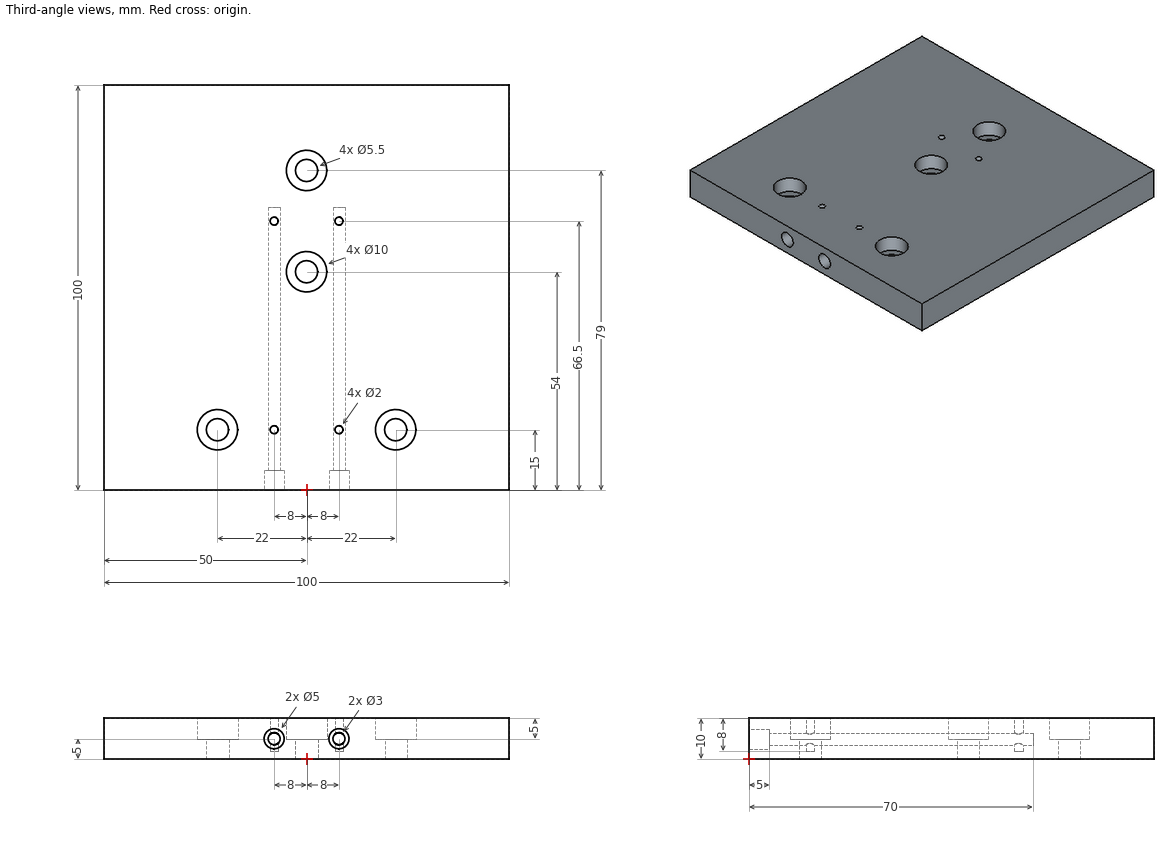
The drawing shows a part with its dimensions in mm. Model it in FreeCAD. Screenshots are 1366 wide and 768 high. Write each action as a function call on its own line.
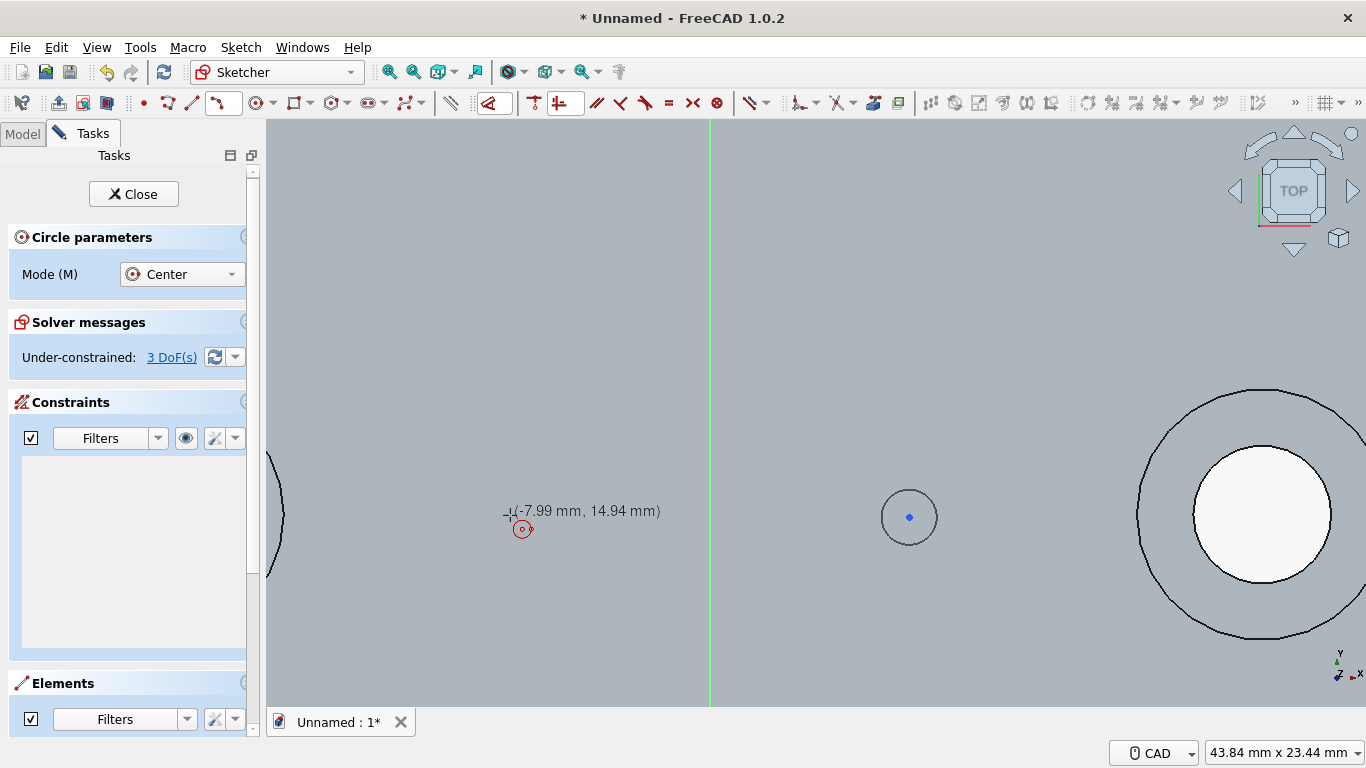
scroll(757, 506, down, 8)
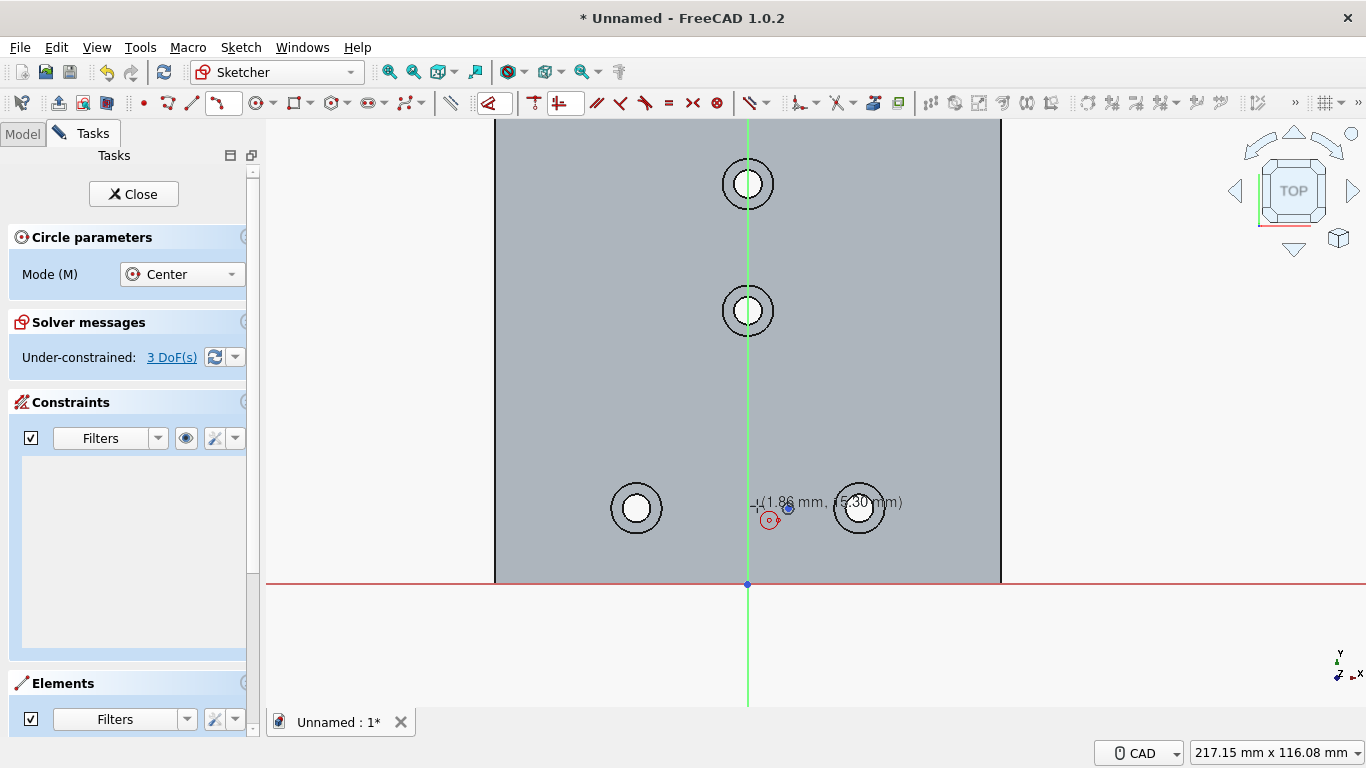
click(707, 508)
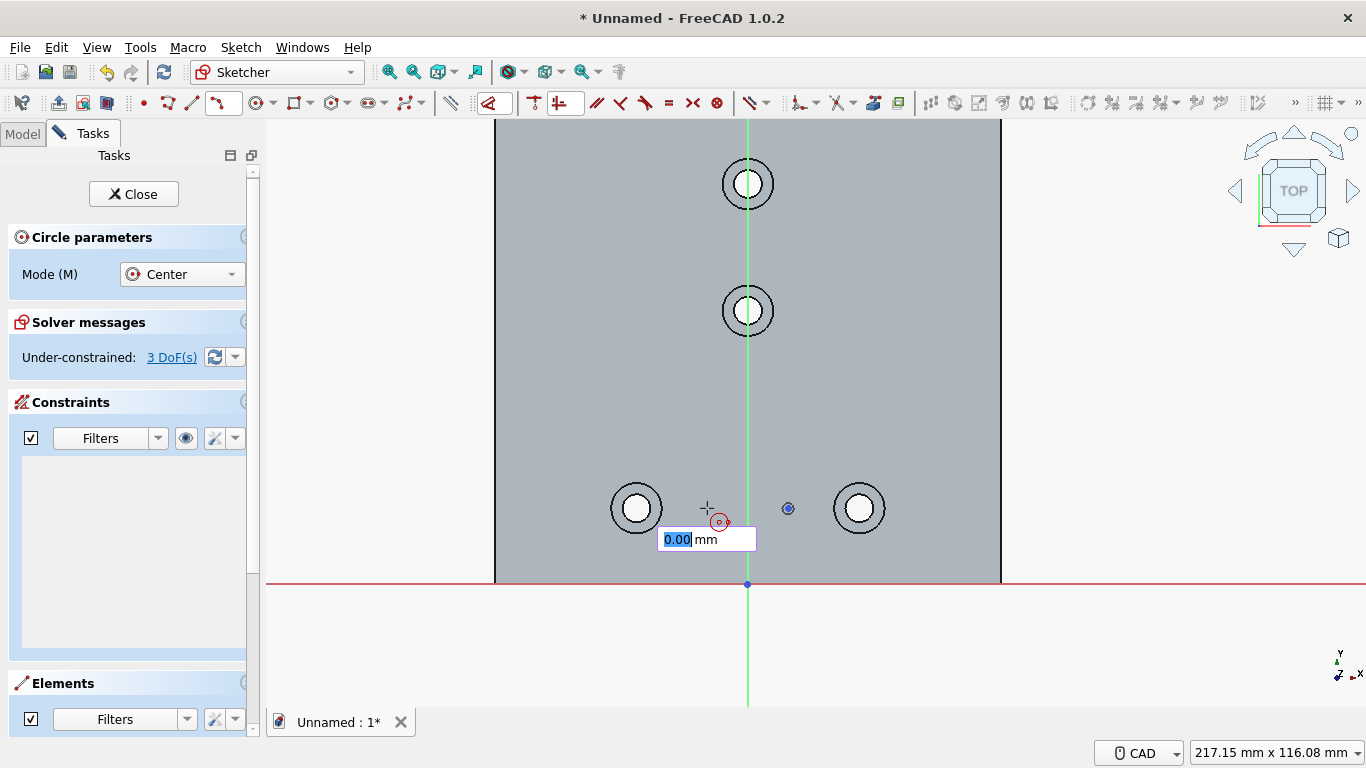
scroll(711, 505, up, 6)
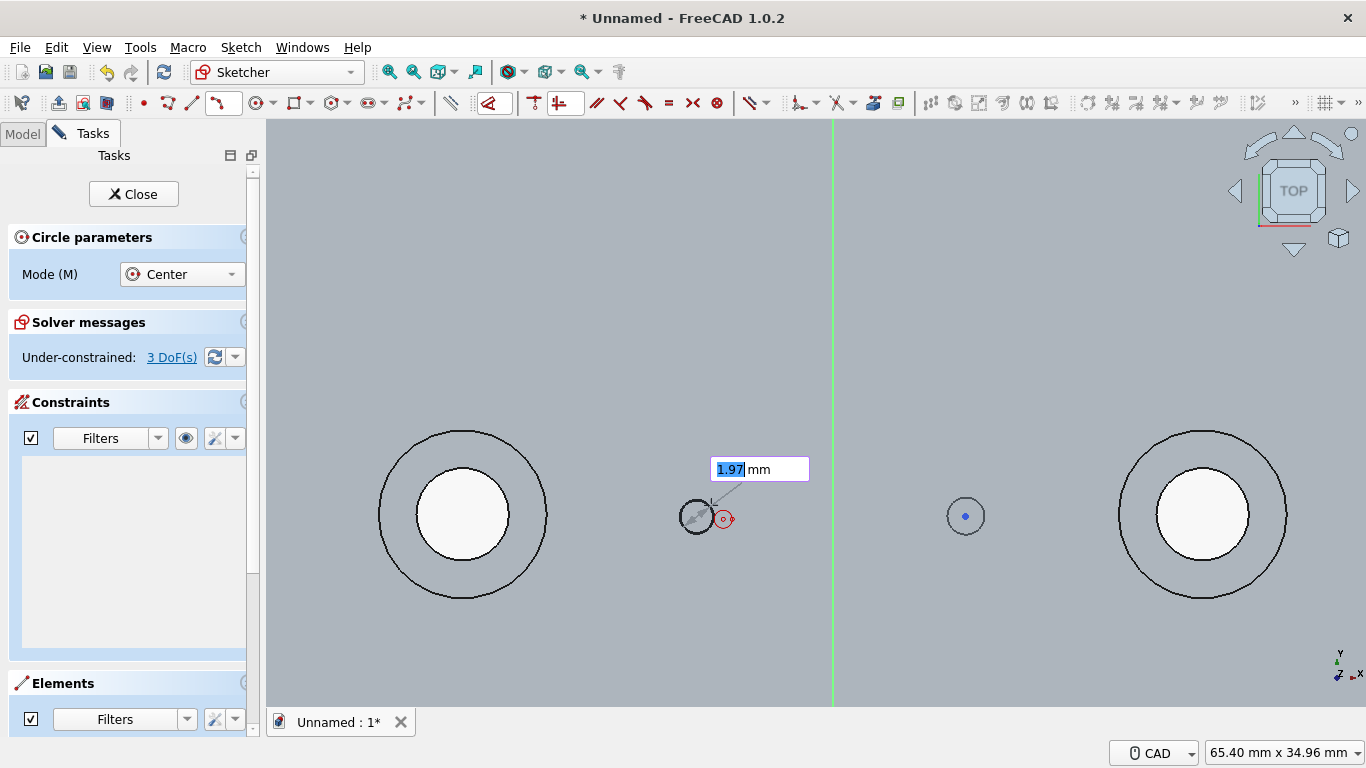
click(710, 502)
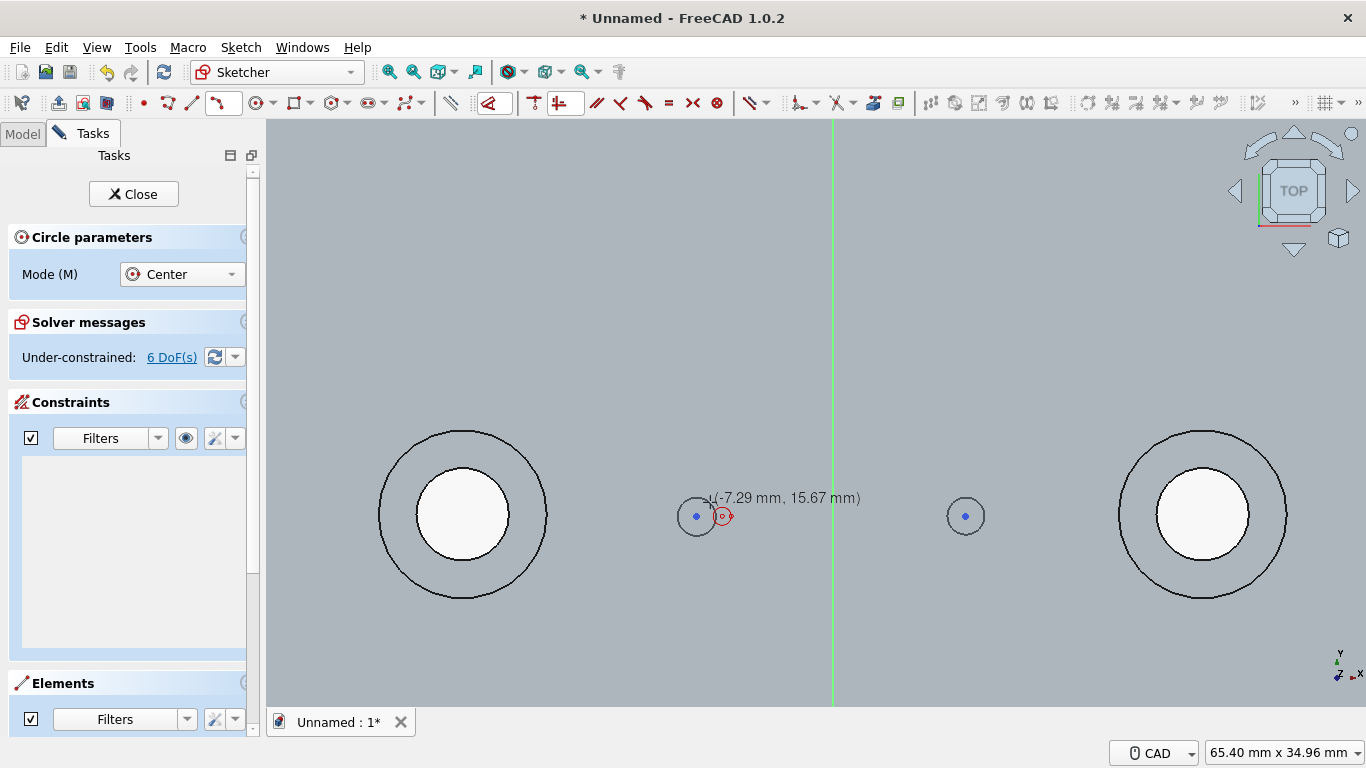
scroll(711, 505, down, 6)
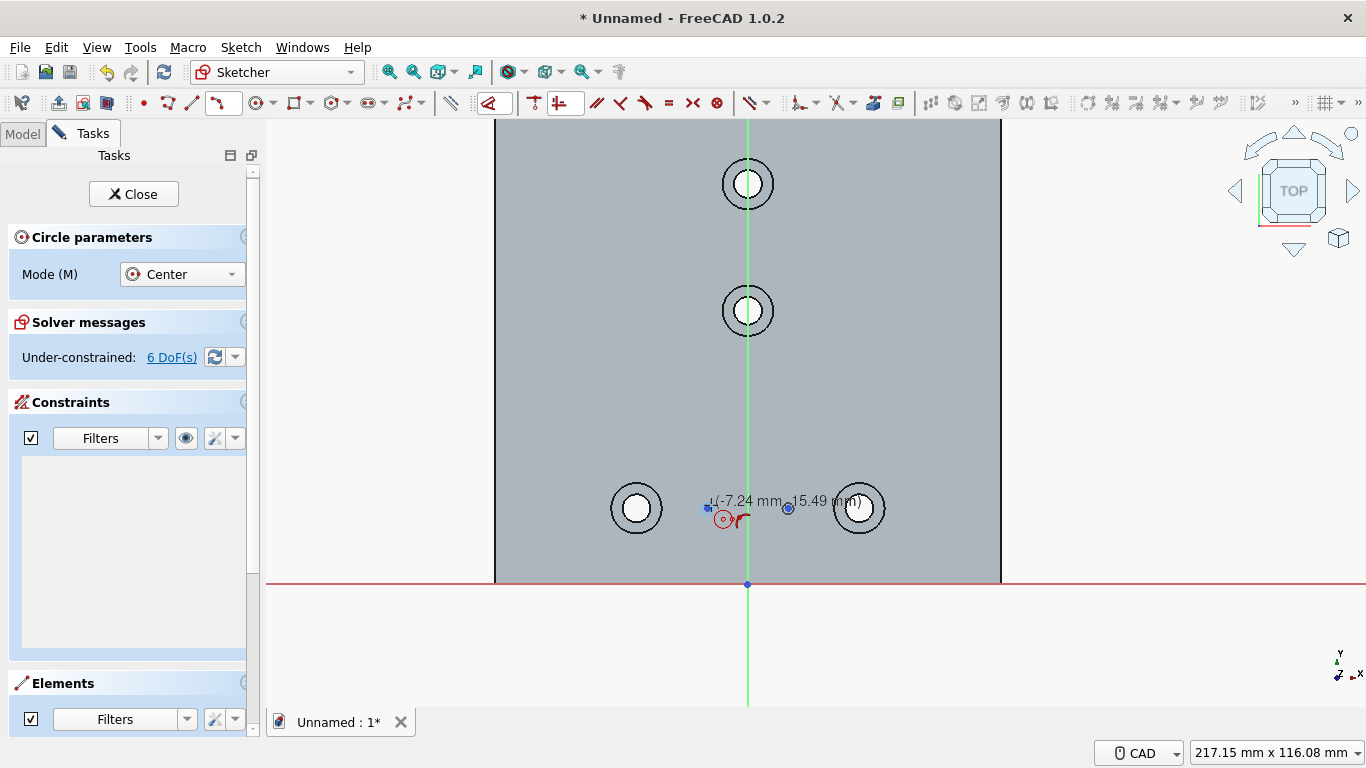
scroll(788, 247, up, 8)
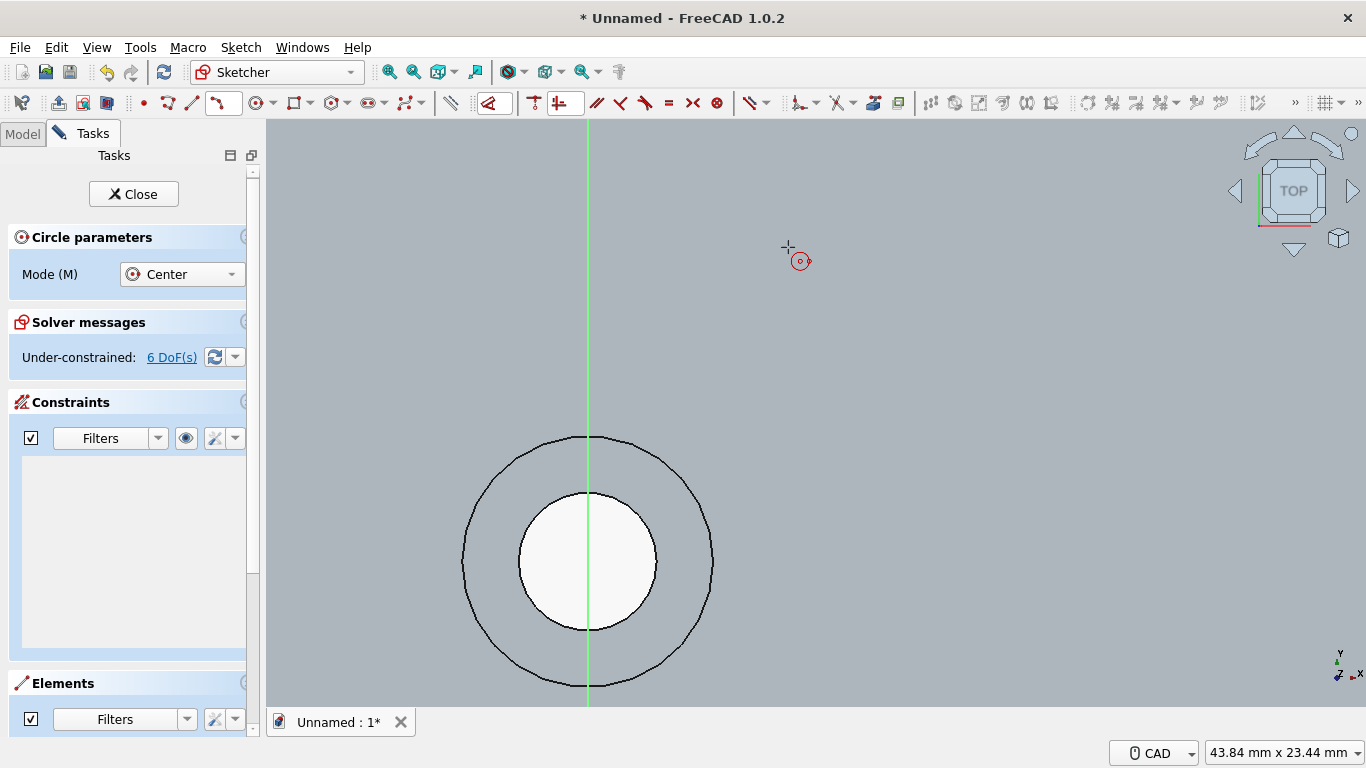
scroll(788, 247, down, 8)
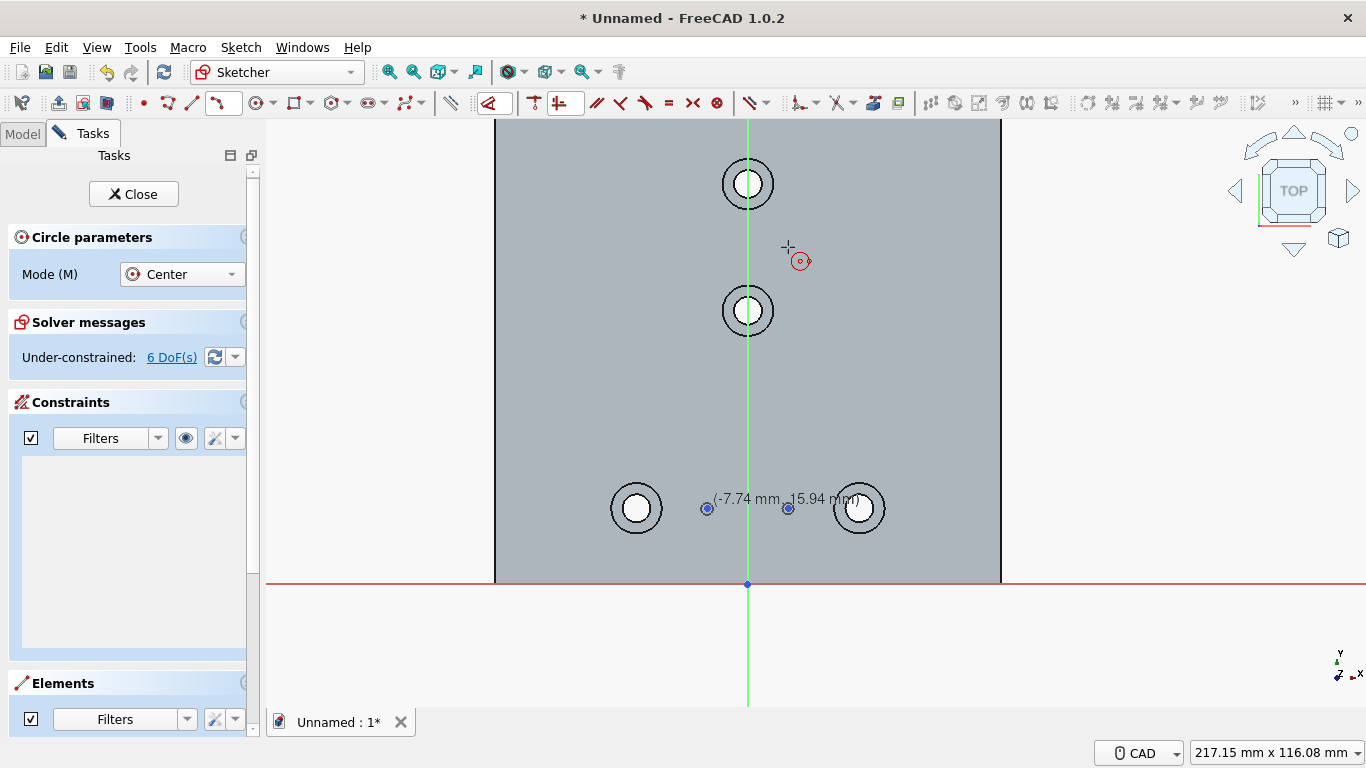
click(788, 247)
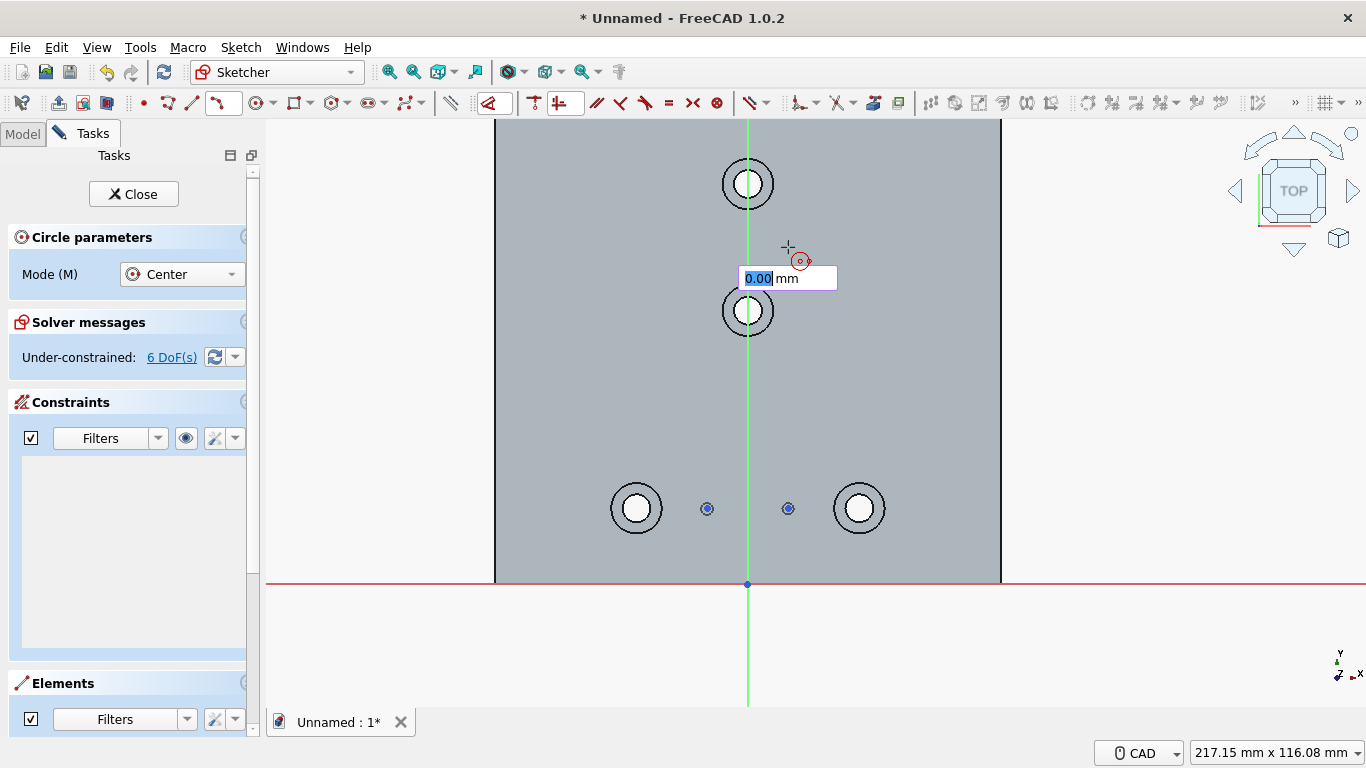
scroll(792, 244, up, 6)